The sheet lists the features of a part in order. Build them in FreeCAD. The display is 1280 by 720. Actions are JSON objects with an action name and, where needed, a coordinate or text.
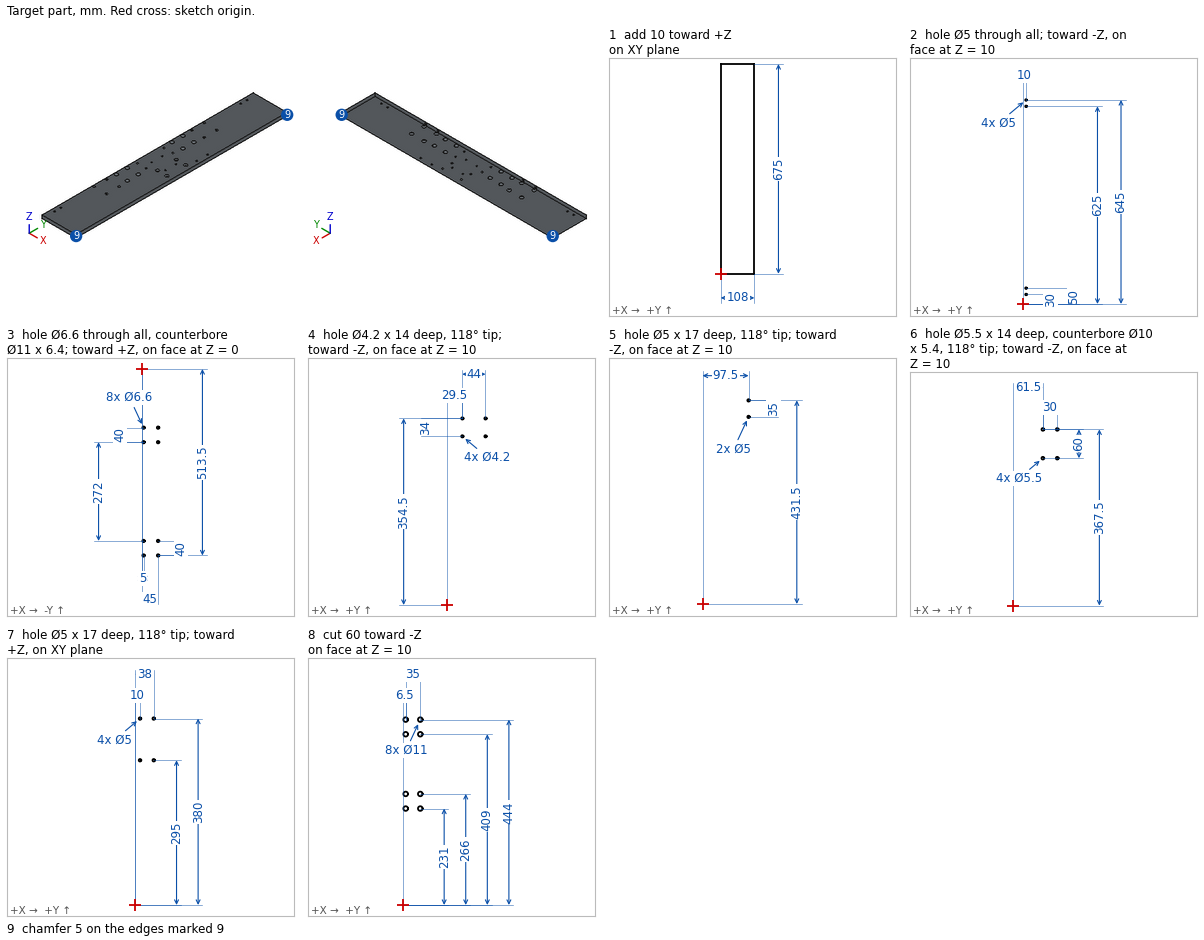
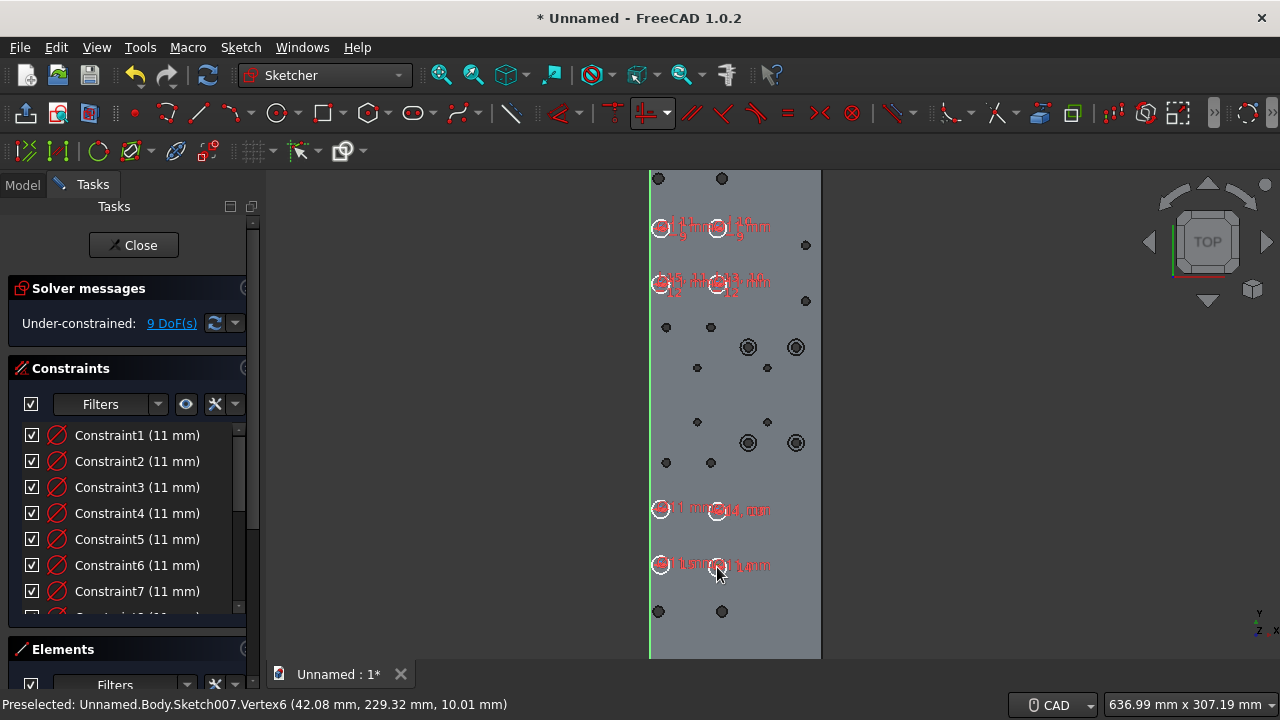
{"action": "left_click", "coordinate": [661, 565]}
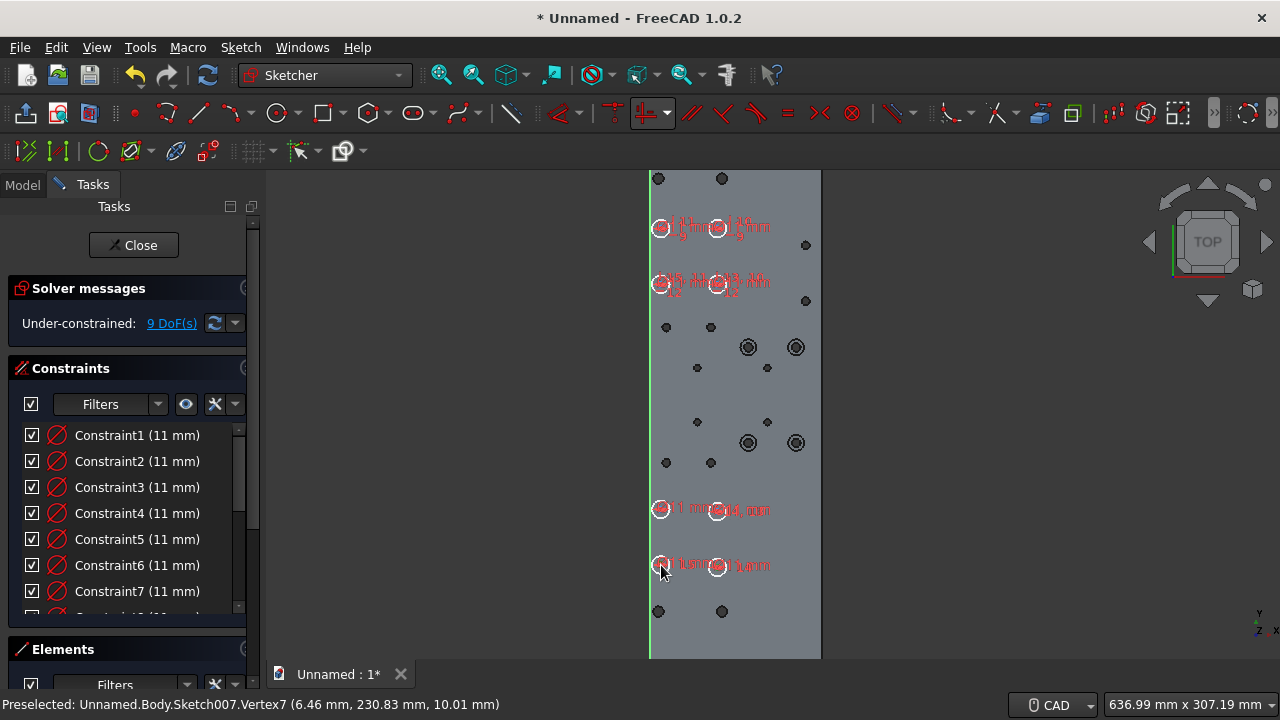
{"action": "key", "text": "h"}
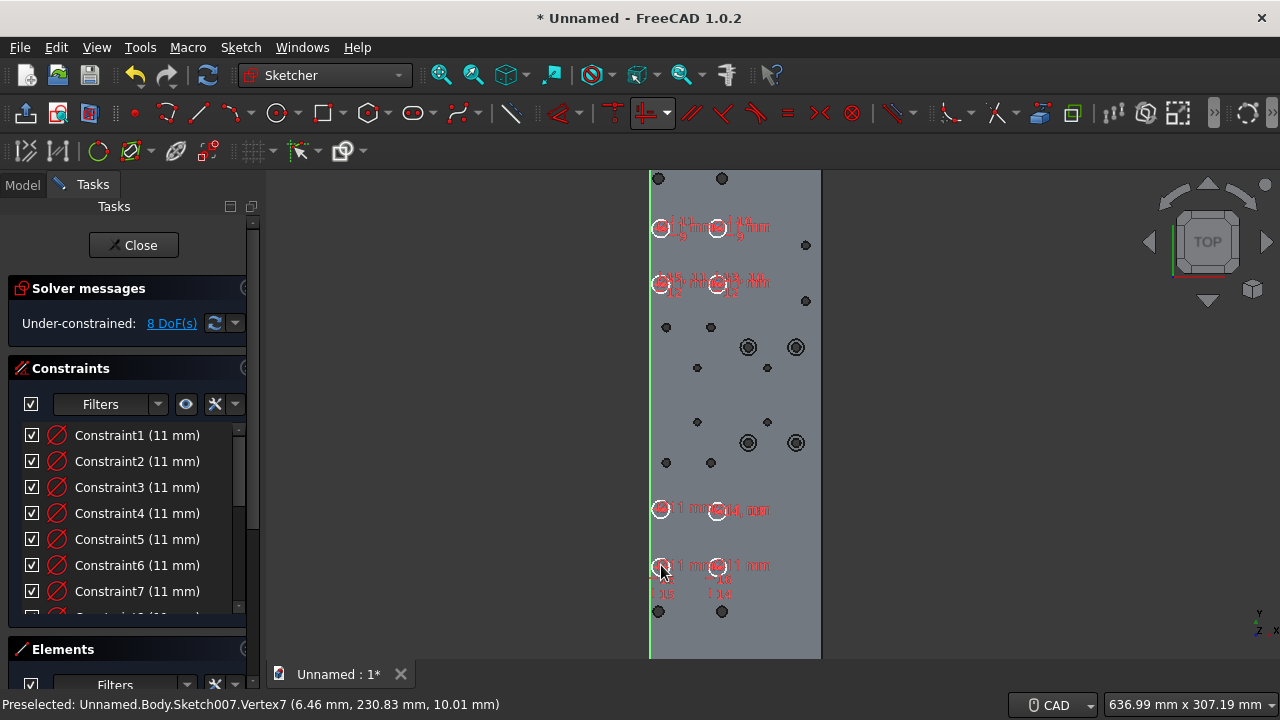
{"action": "left_click", "coordinate": [661, 567]}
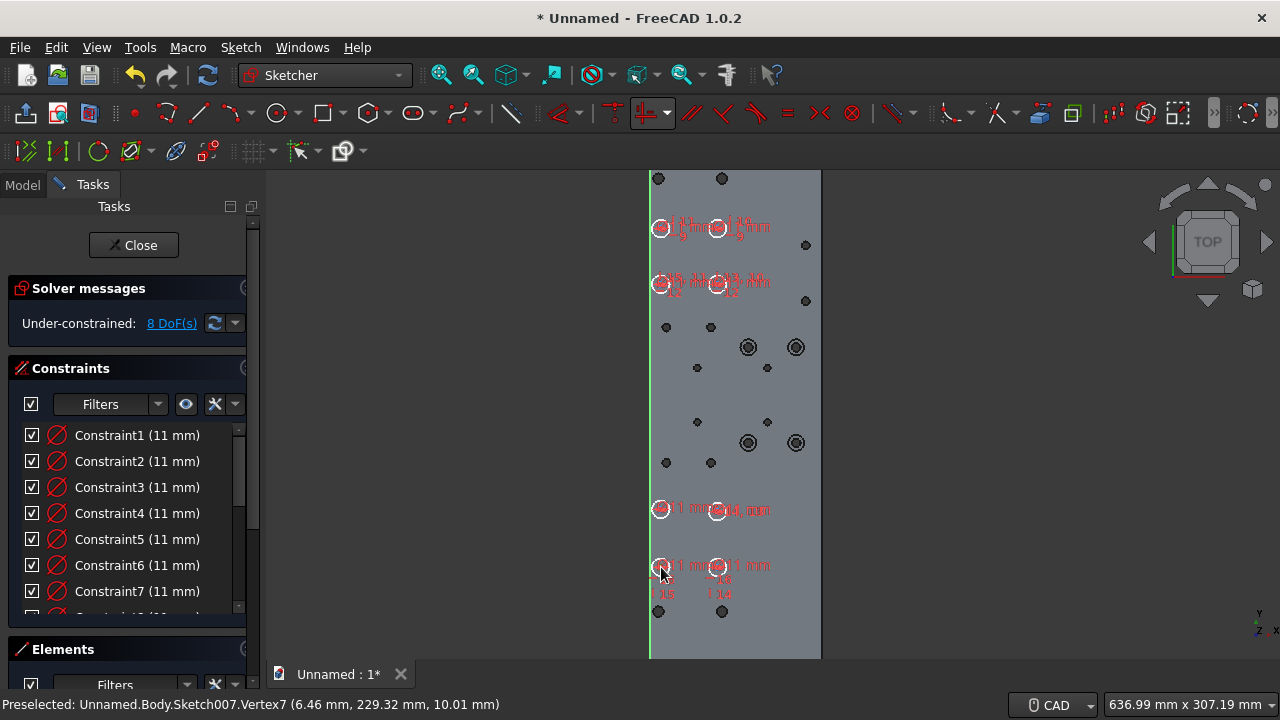
{"action": "left_click", "coordinate": [661, 509]}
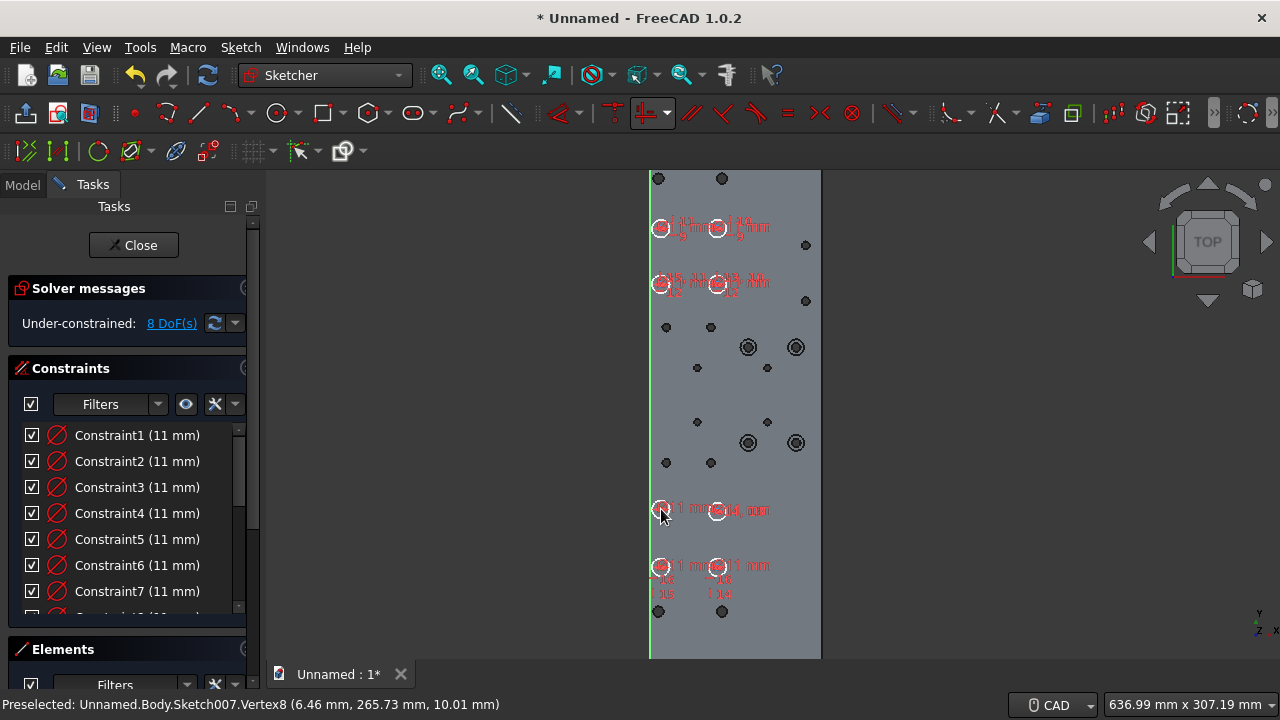
{"action": "key", "text": "v"}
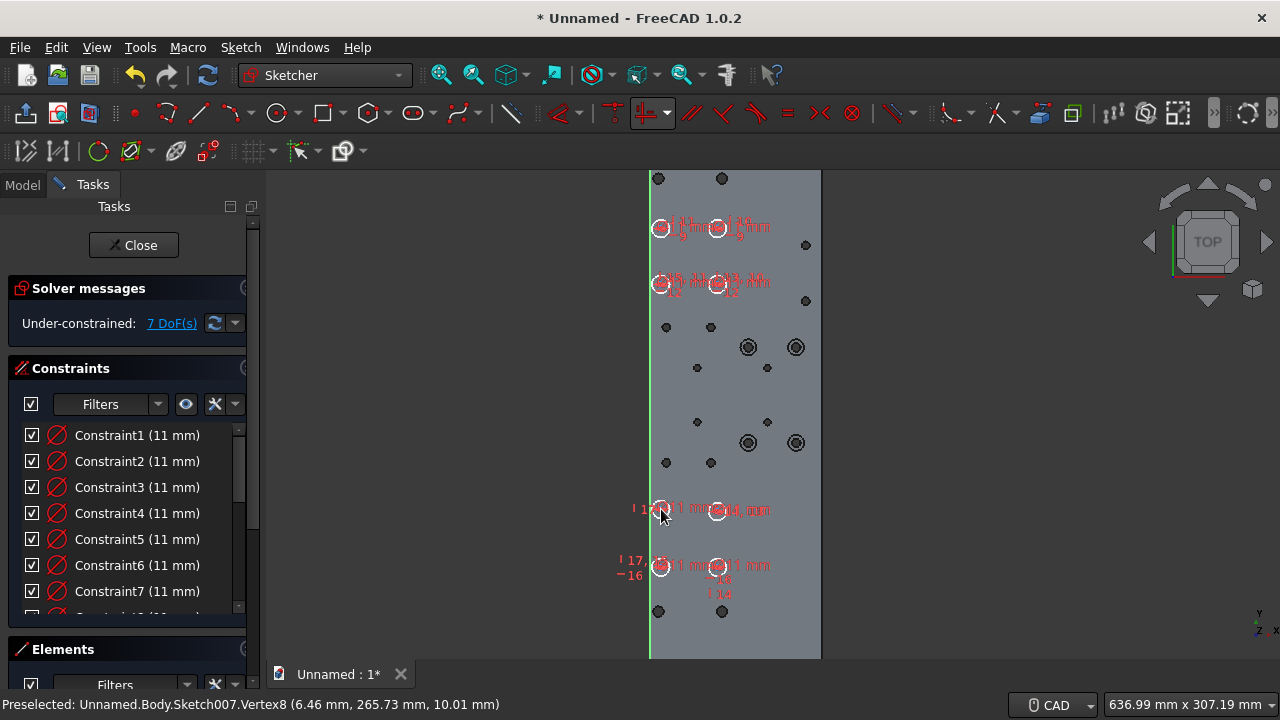
{"action": "left_click", "coordinate": [717, 512]}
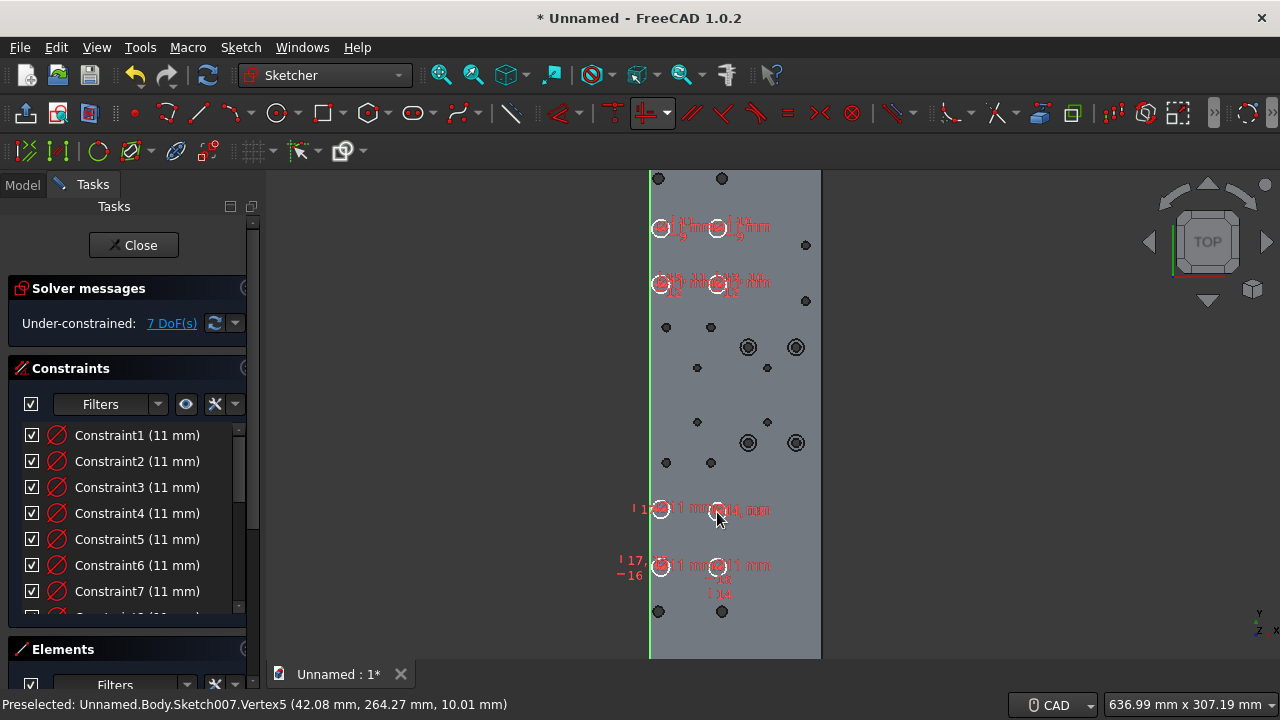
{"action": "left_click", "coordinate": [661, 509]}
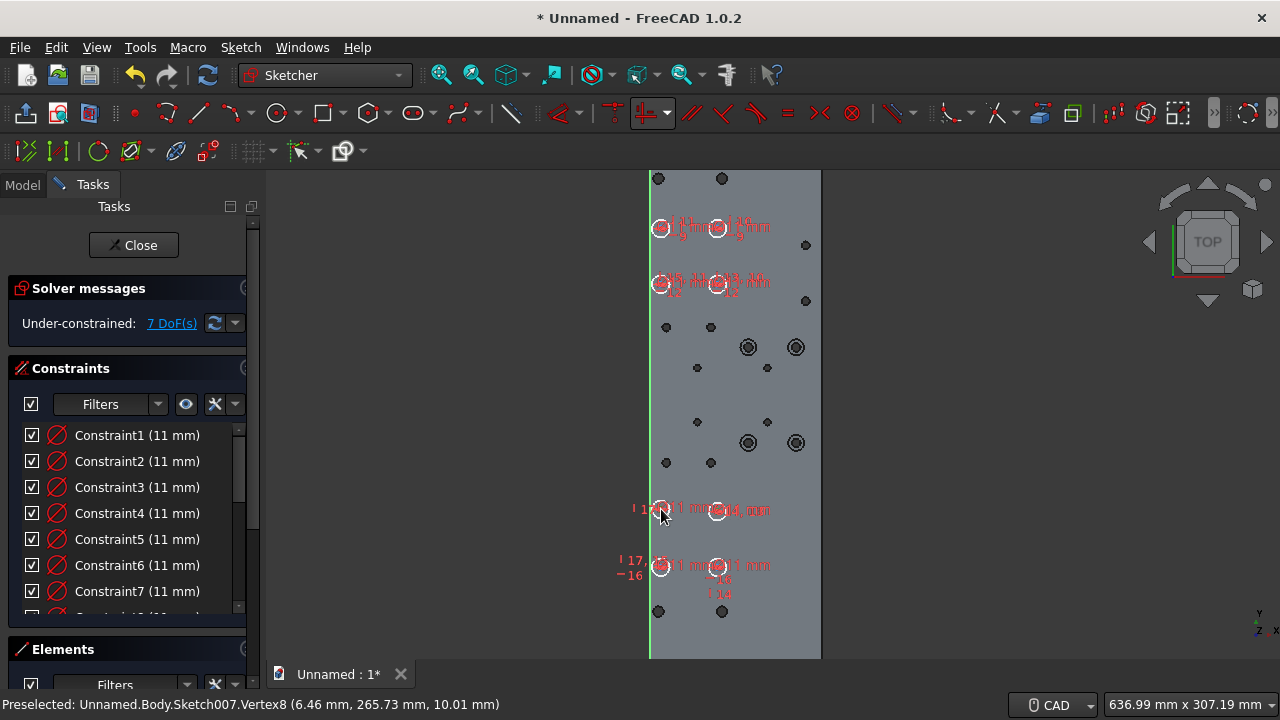
{"action": "key", "text": "h"}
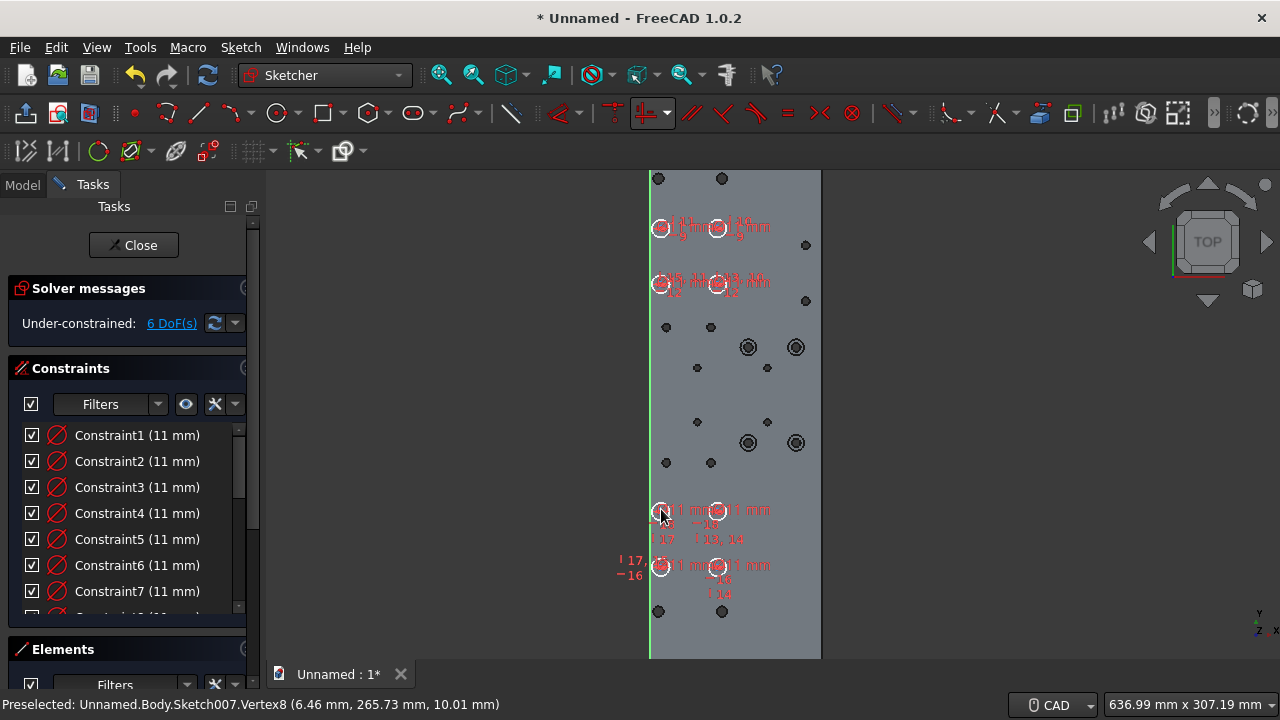
{"action": "left_click", "coordinate": [558, 114]}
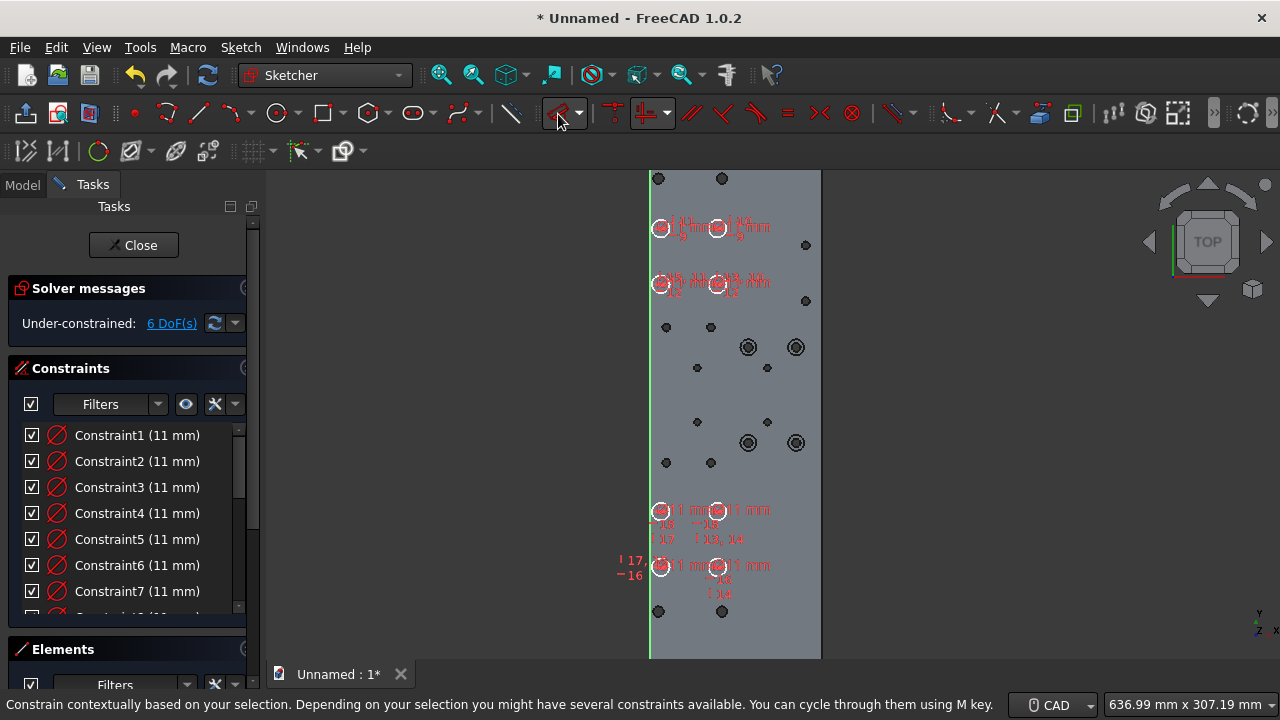
{"action": "left_click", "coordinate": [717, 229]}
{"action": "left_click", "coordinate": [616, 430]}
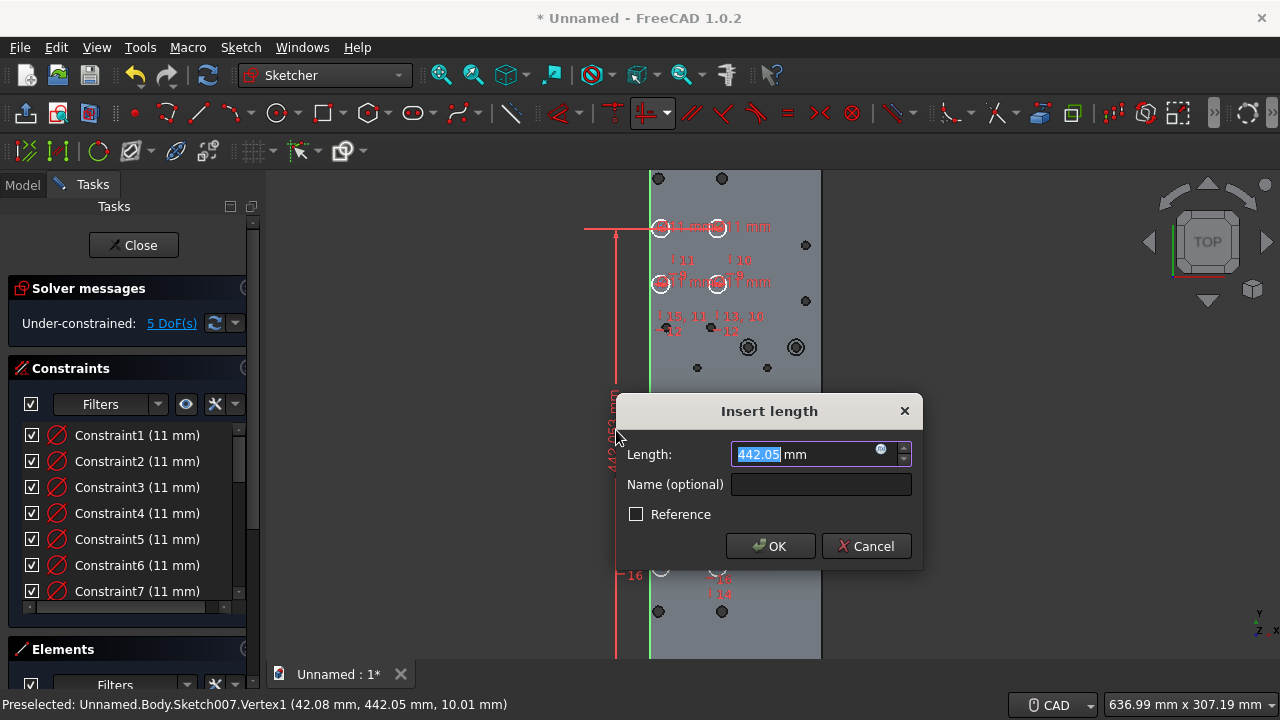
{"action": "type", "text": "444"}
{"action": "key", "text": "Return"}